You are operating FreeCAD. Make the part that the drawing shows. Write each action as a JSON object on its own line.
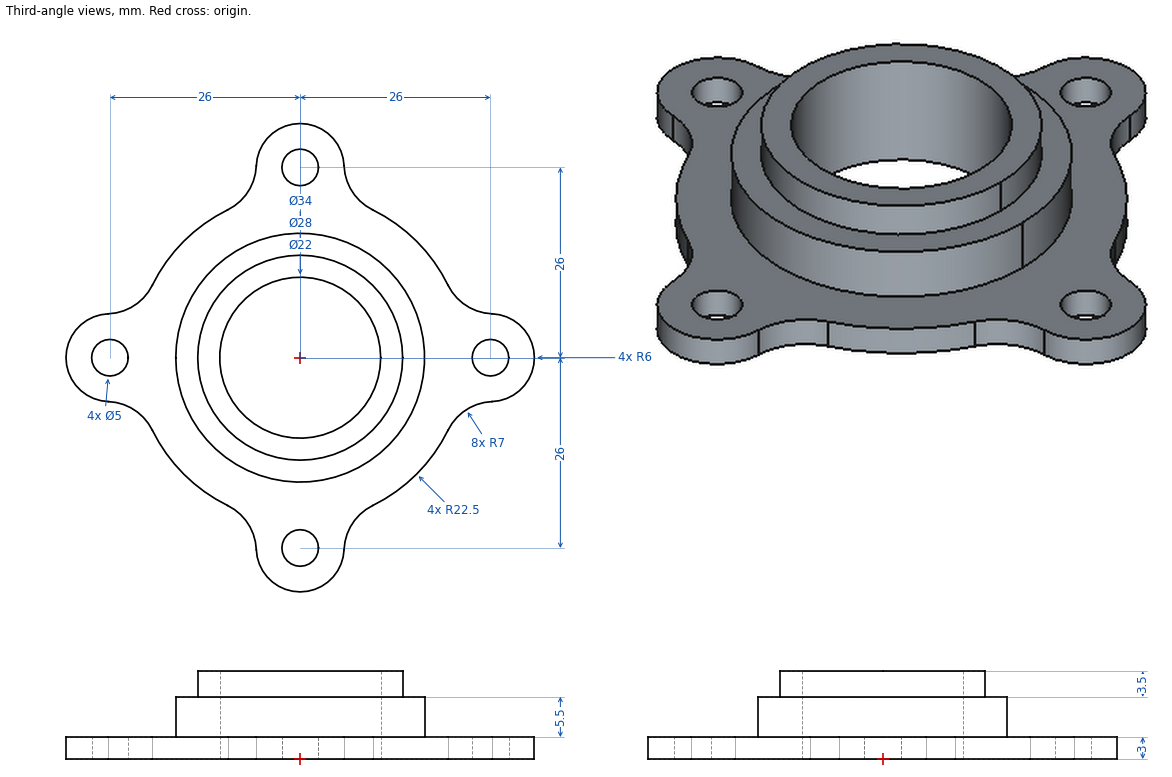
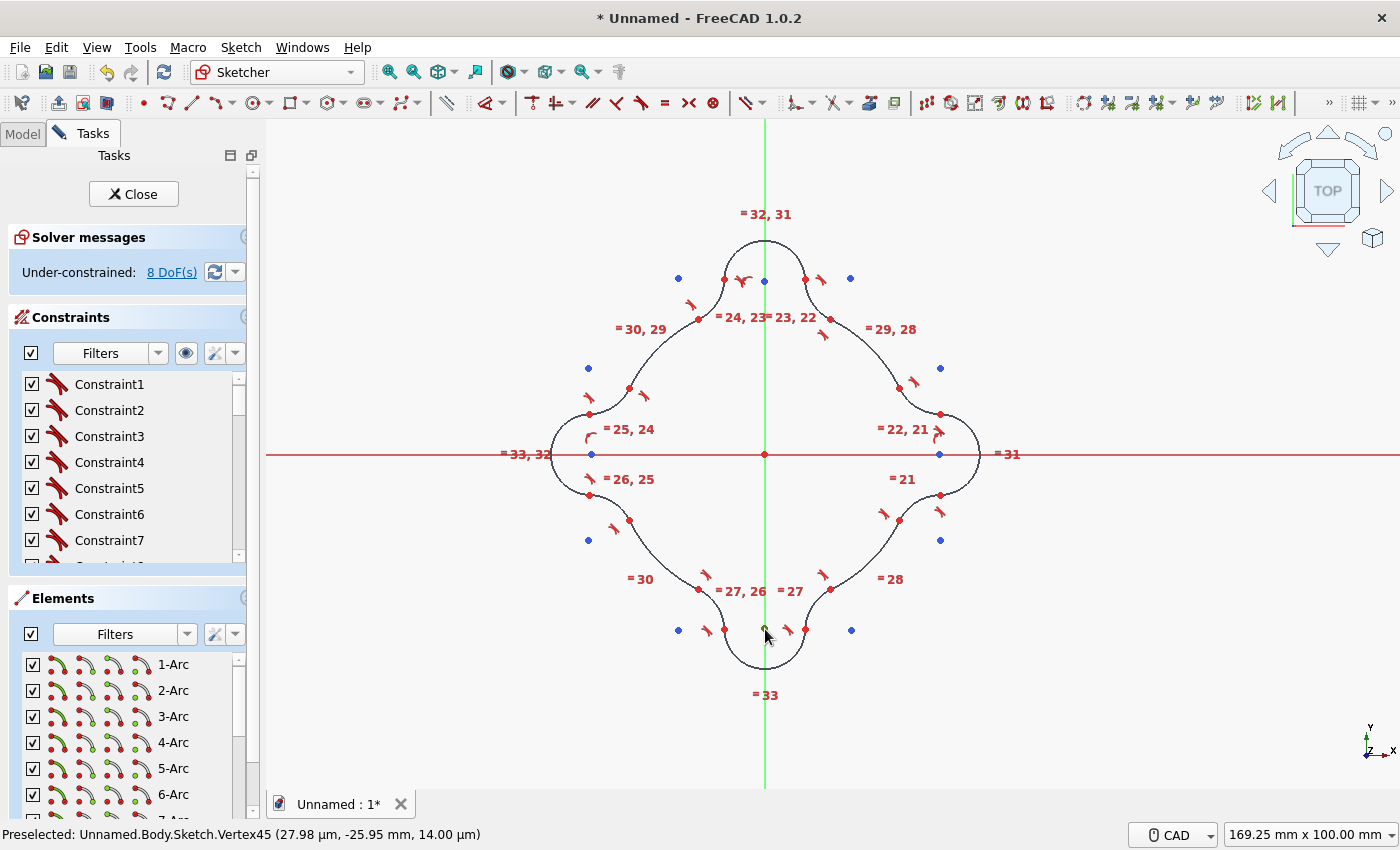
{"action": "left_click", "coordinate": [765, 717]}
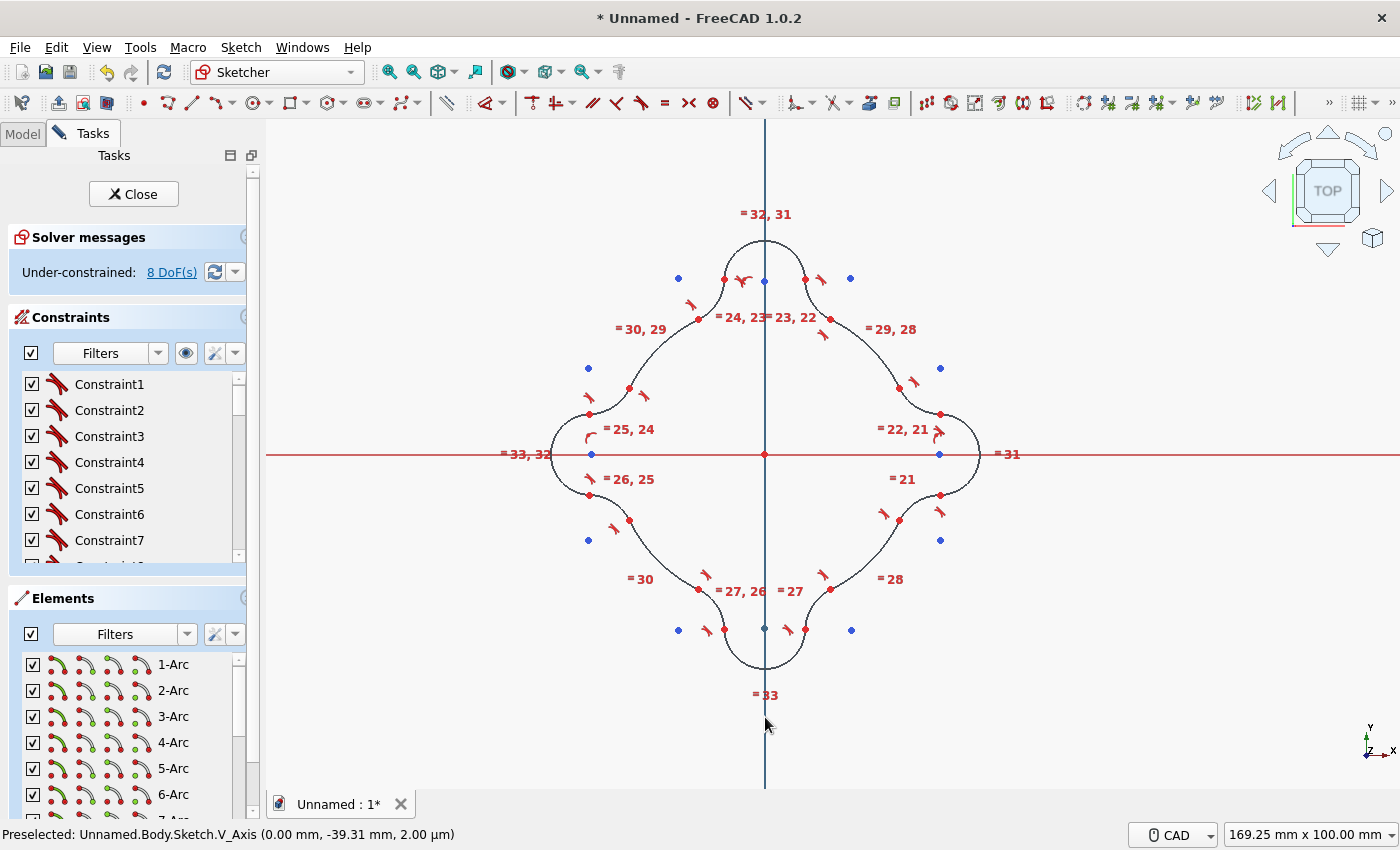
{"action": "left_click", "coordinate": [532, 104]}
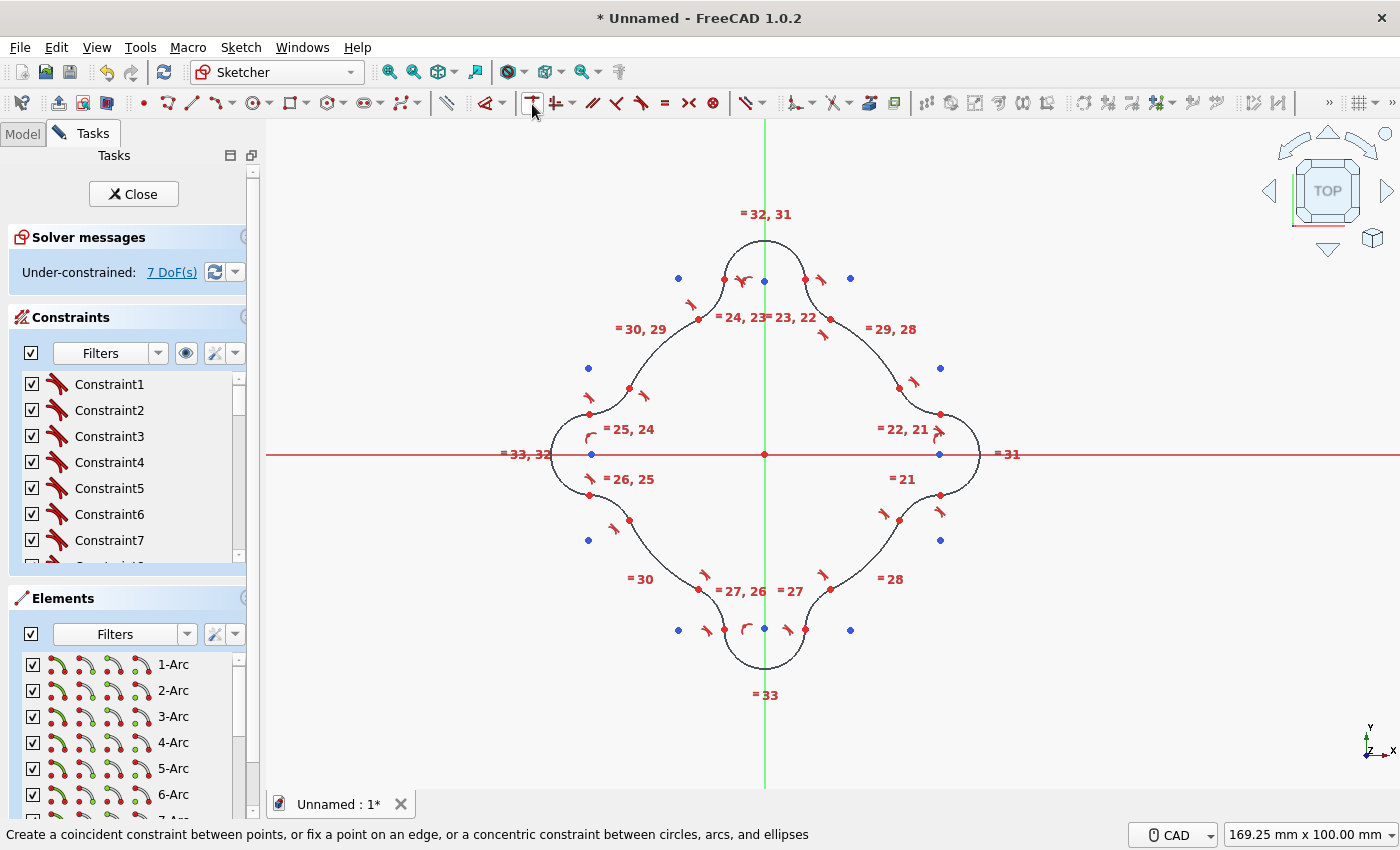
{"action": "left_click", "coordinate": [486, 104]}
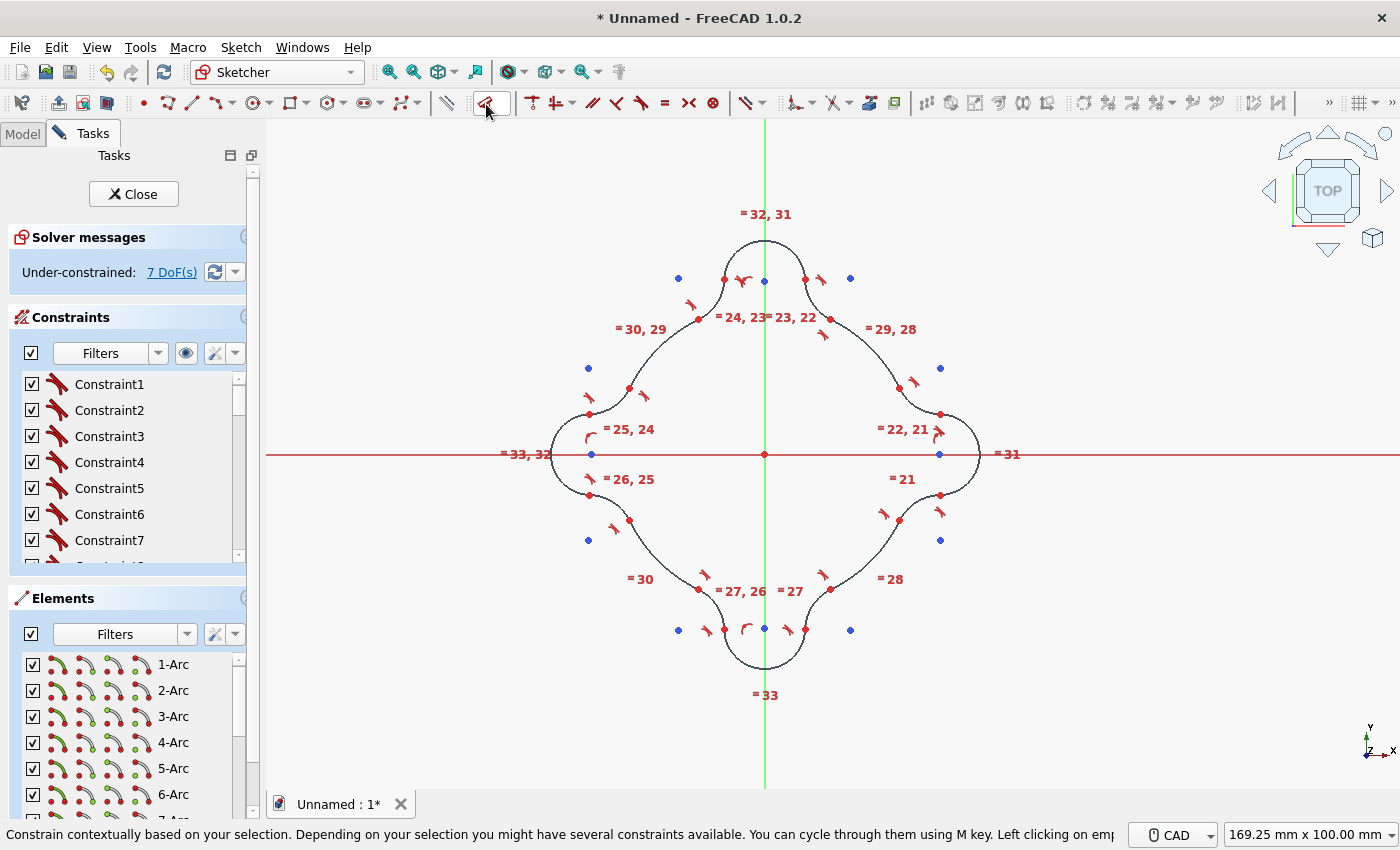
{"action": "left_click", "coordinate": [856, 574]}
{"action": "left_click", "coordinate": [875, 599]}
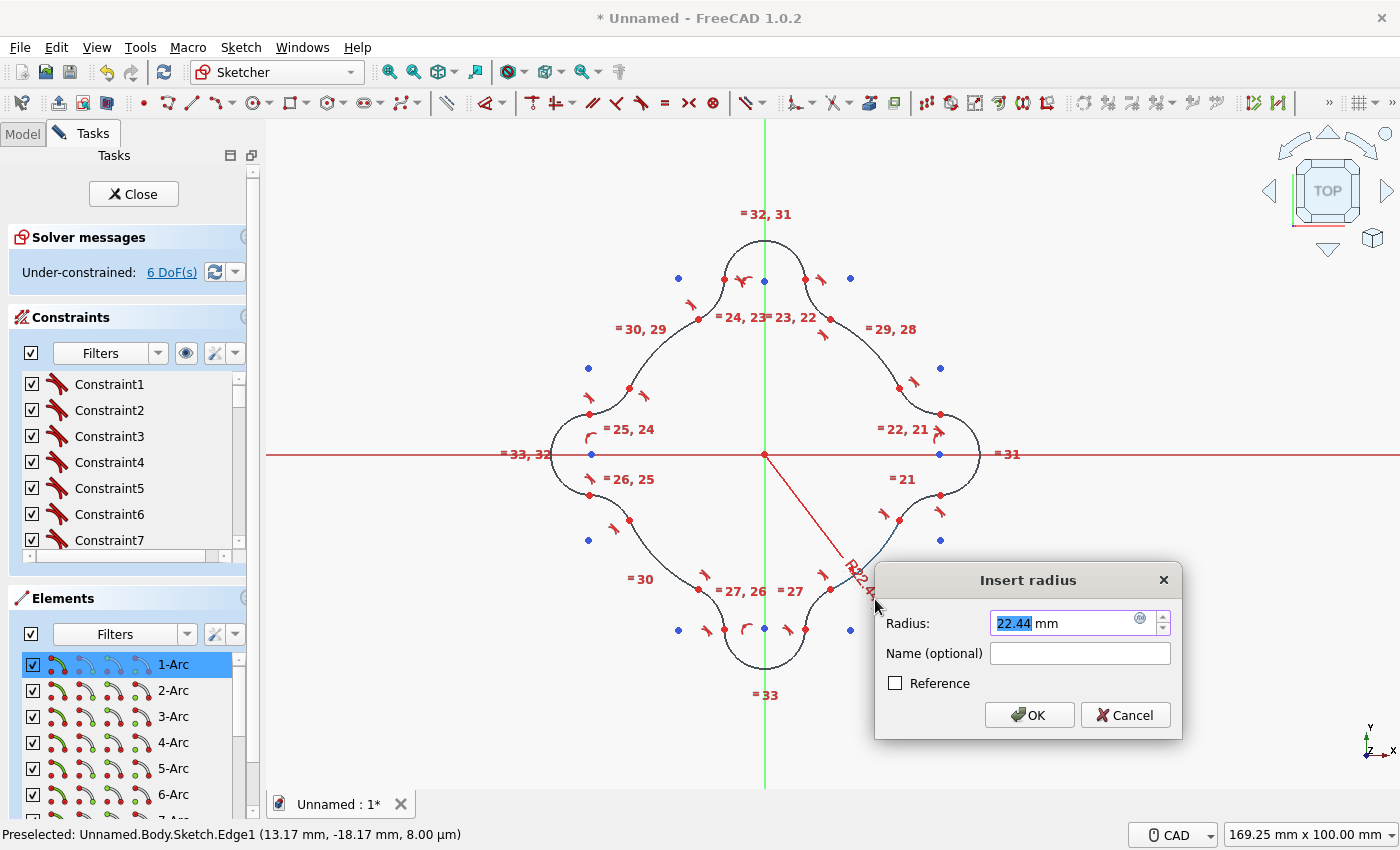
{"action": "type", "text": "22.5"}
{"action": "key", "text": "Return"}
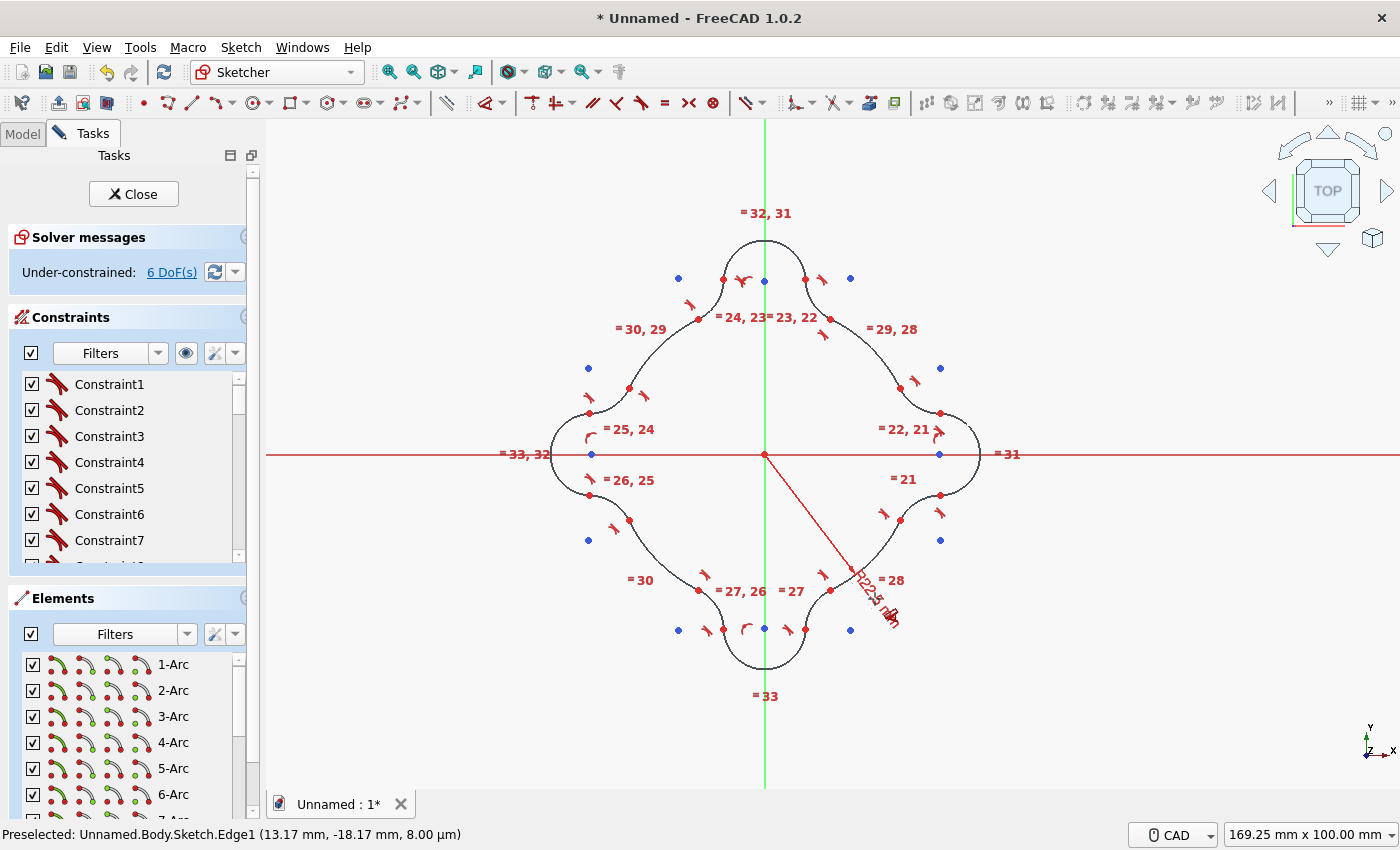
{"action": "left_click", "coordinate": [925, 498]}
{"action": "left_click", "coordinate": [914, 468]}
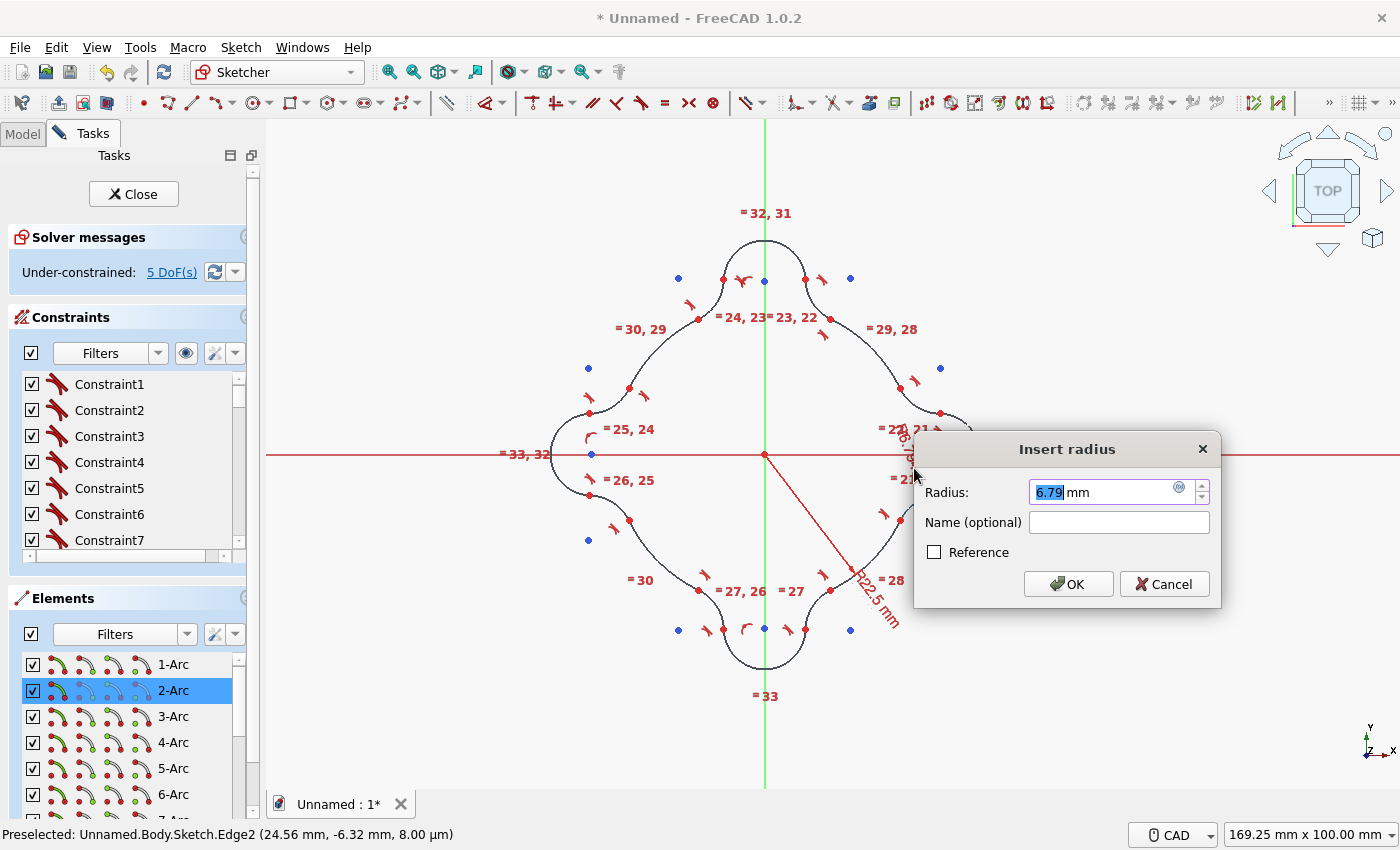
{"action": "type", "text": "7"}
{"action": "key", "text": "Return"}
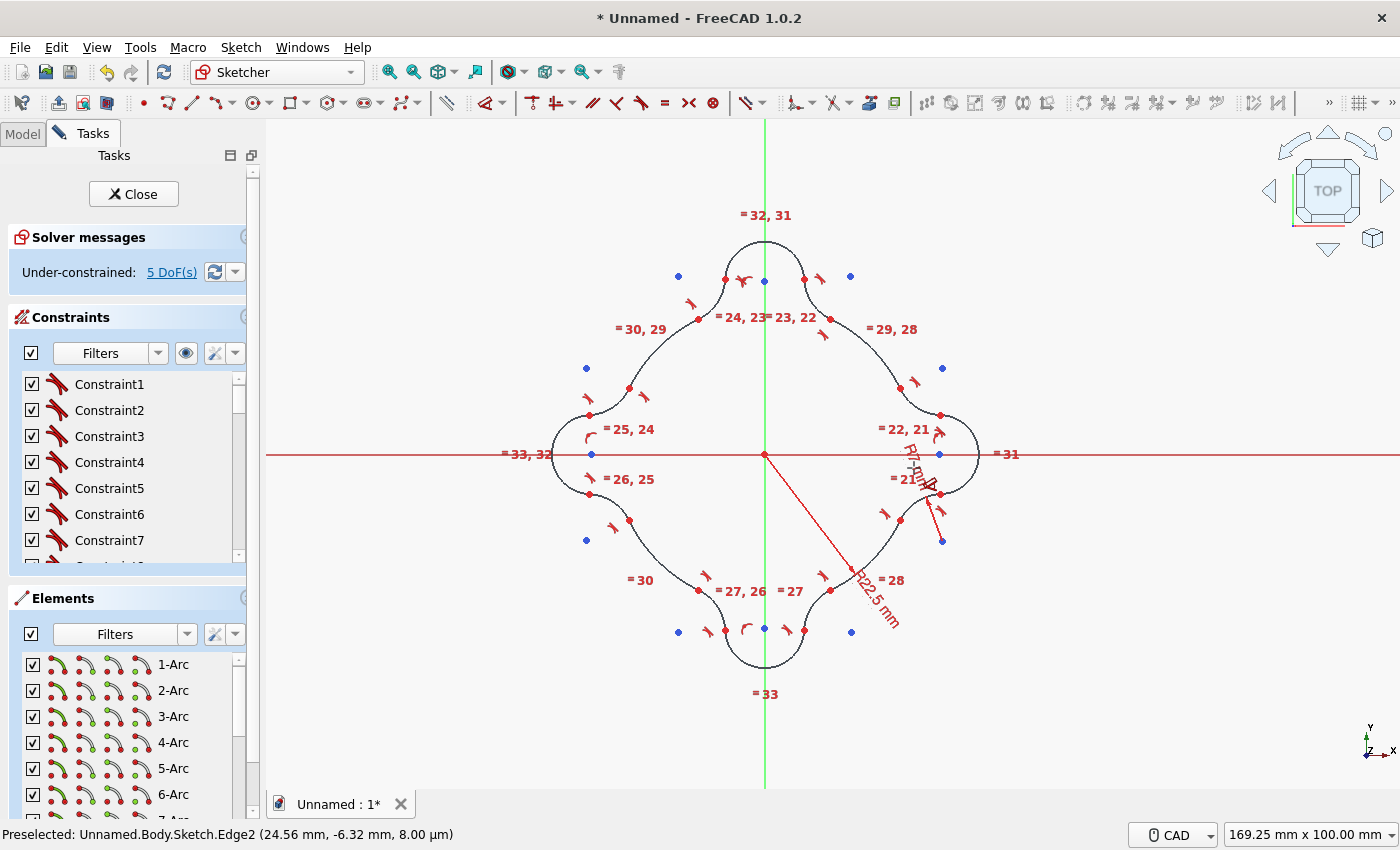
{"action": "left_click", "coordinate": [972, 477]}
{"action": "left_click", "coordinate": [998, 495]}